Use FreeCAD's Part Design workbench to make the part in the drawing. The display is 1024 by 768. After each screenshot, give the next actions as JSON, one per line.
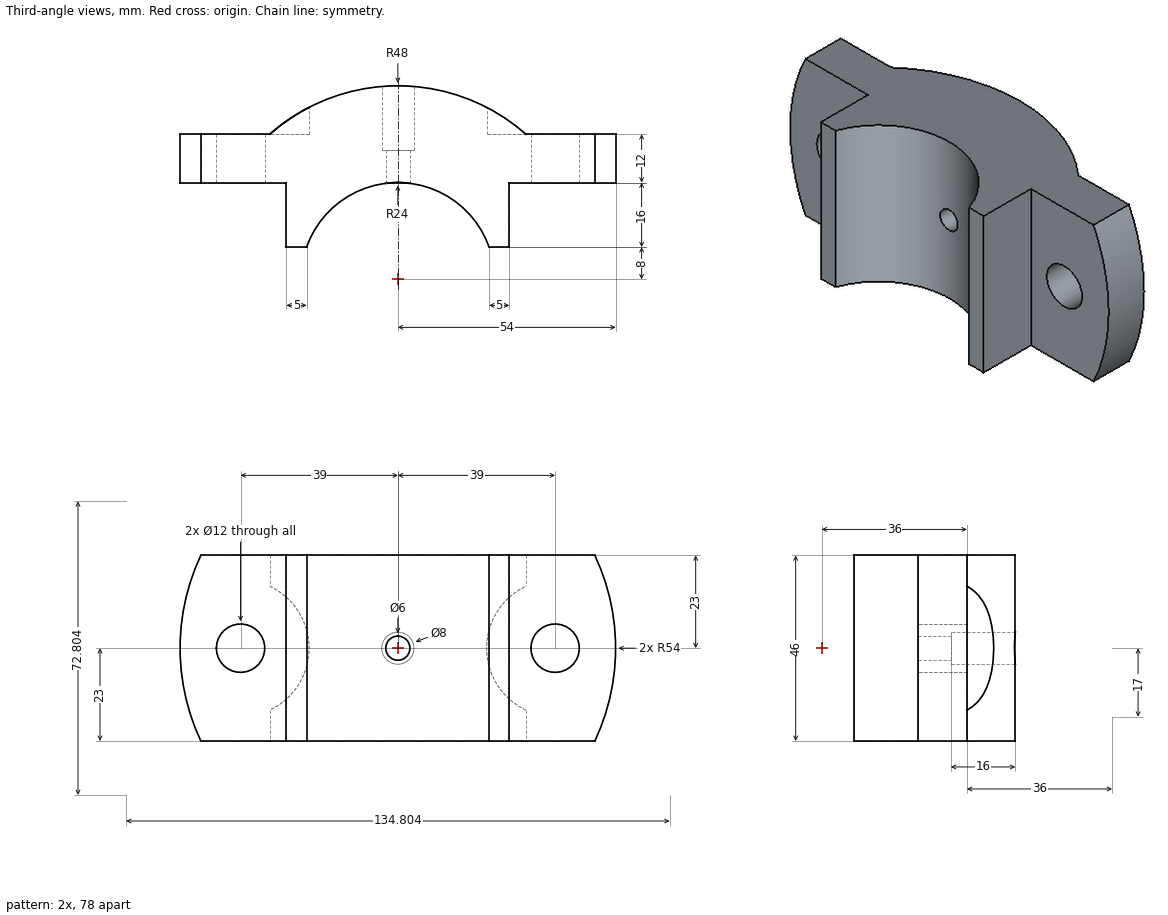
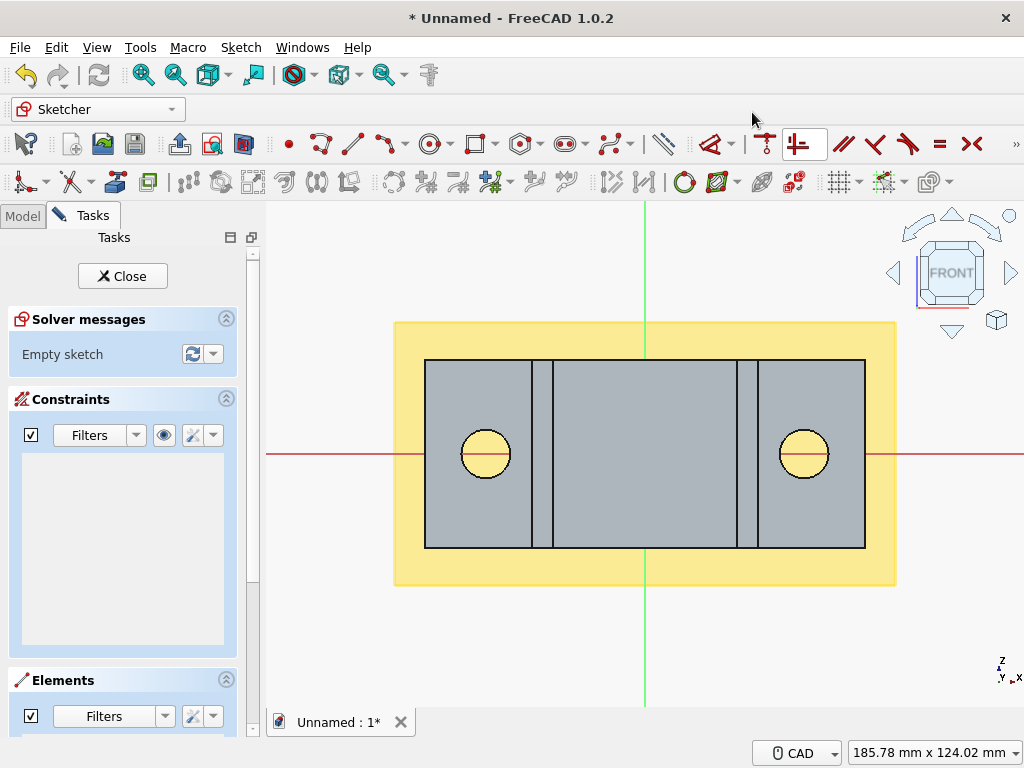
{"action": "left_click", "coordinate": [244, 144]}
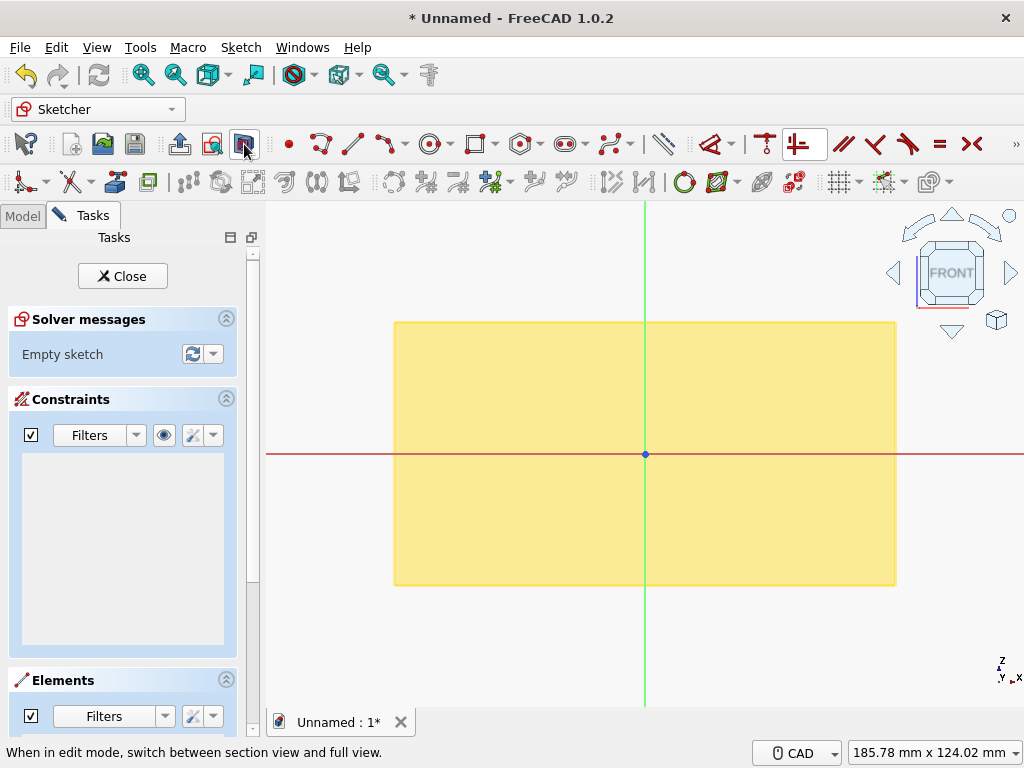
{"action": "scroll", "coordinate": [650, 454], "scroll_direction": "up", "scroll_amount": 13}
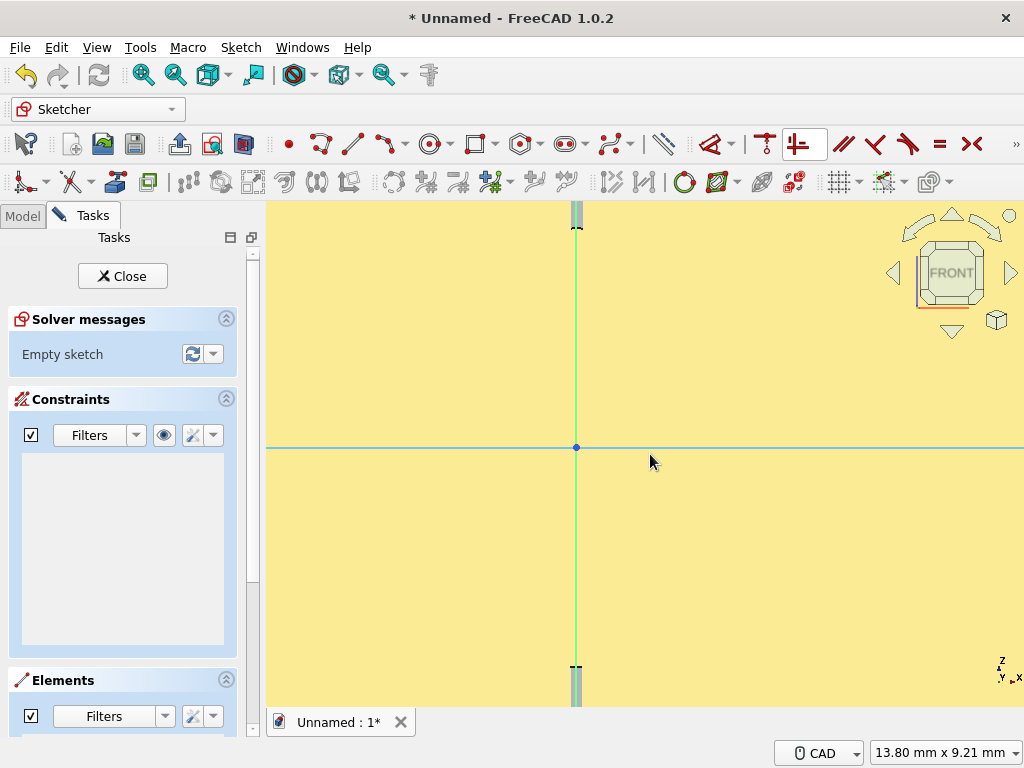
{"action": "left_click", "coordinate": [430, 144]}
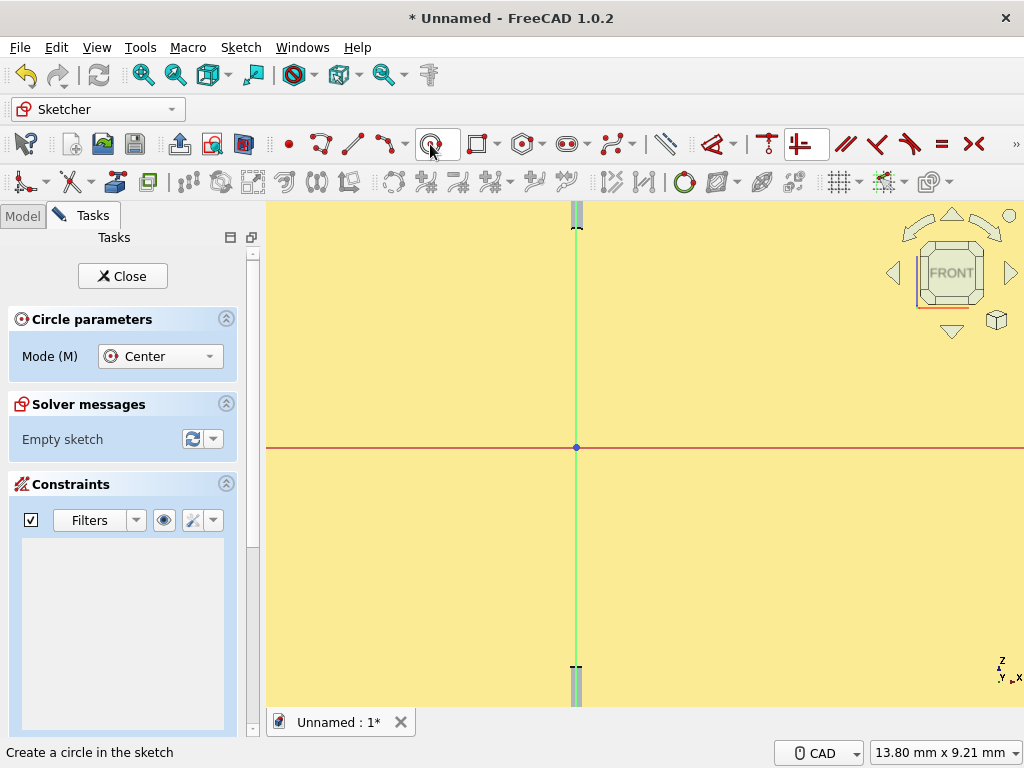
{"action": "left_click", "coordinate": [576, 448]}
{"action": "mouse_move", "coordinate": [693, 331]}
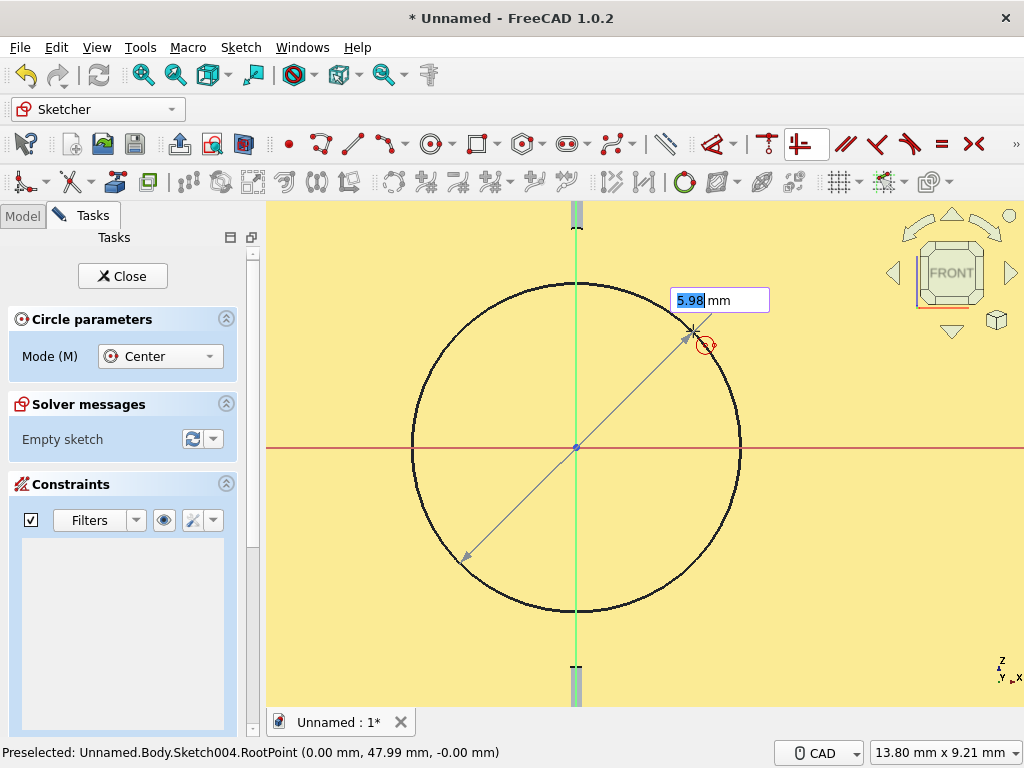
{"action": "type", "text": "6"}
{"action": "key", "text": "Return"}
{"action": "key", "text": "Escape"}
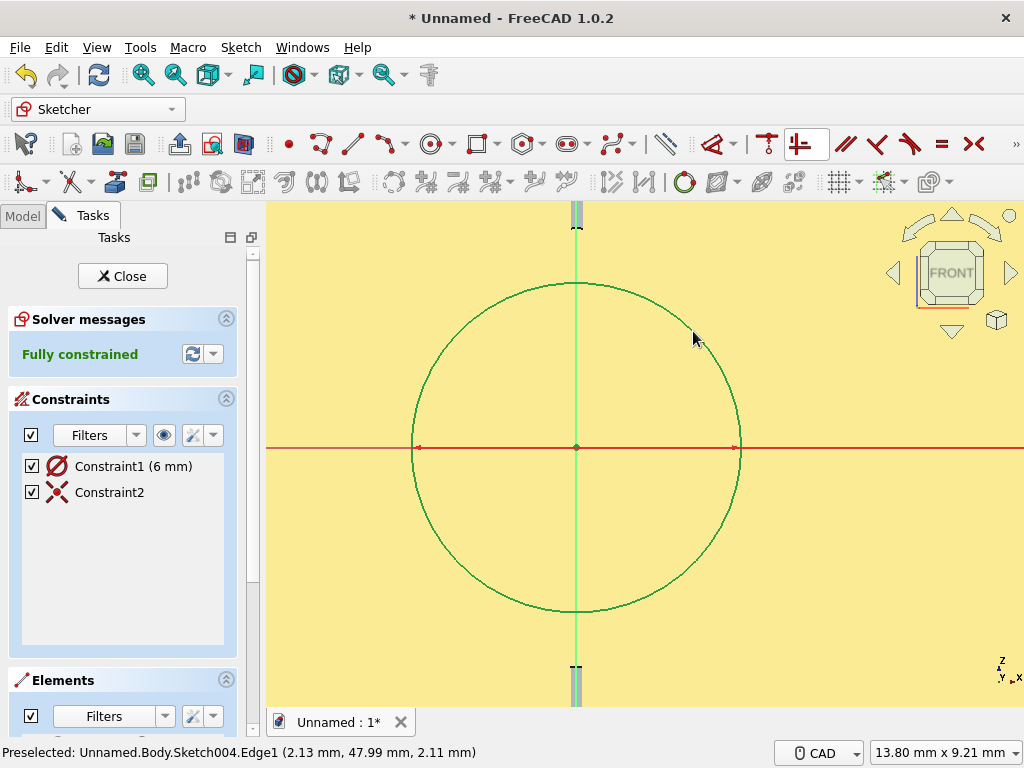
{"action": "left_click", "coordinate": [123, 276]}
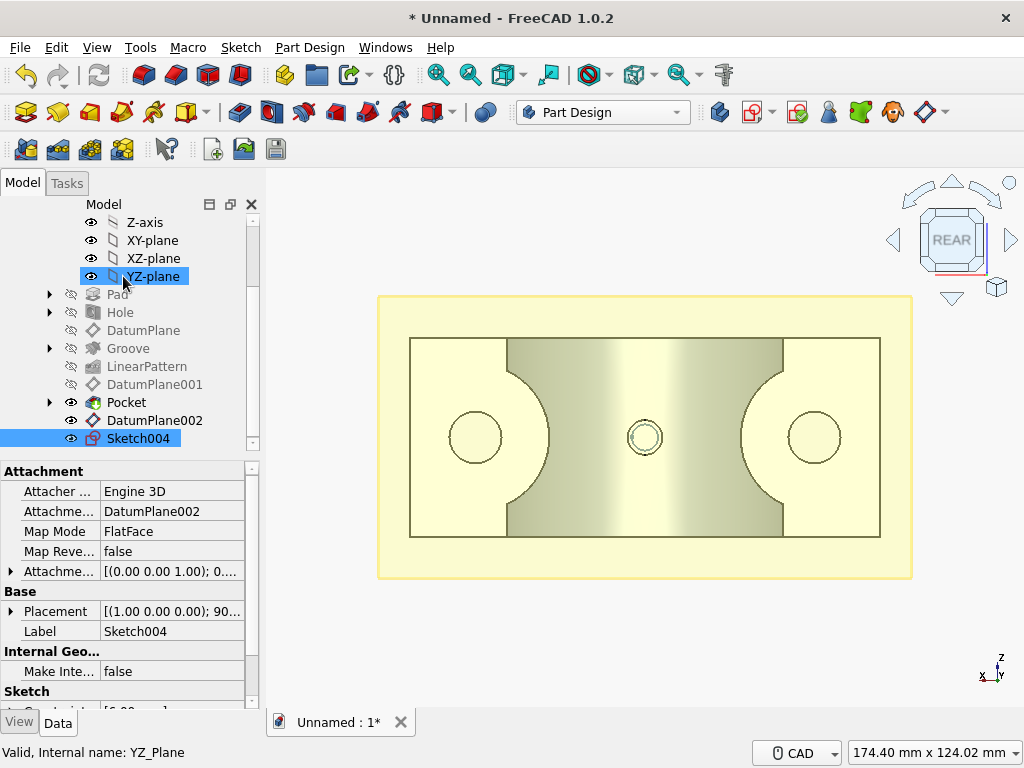
{"action": "left_click", "coordinate": [240, 112]}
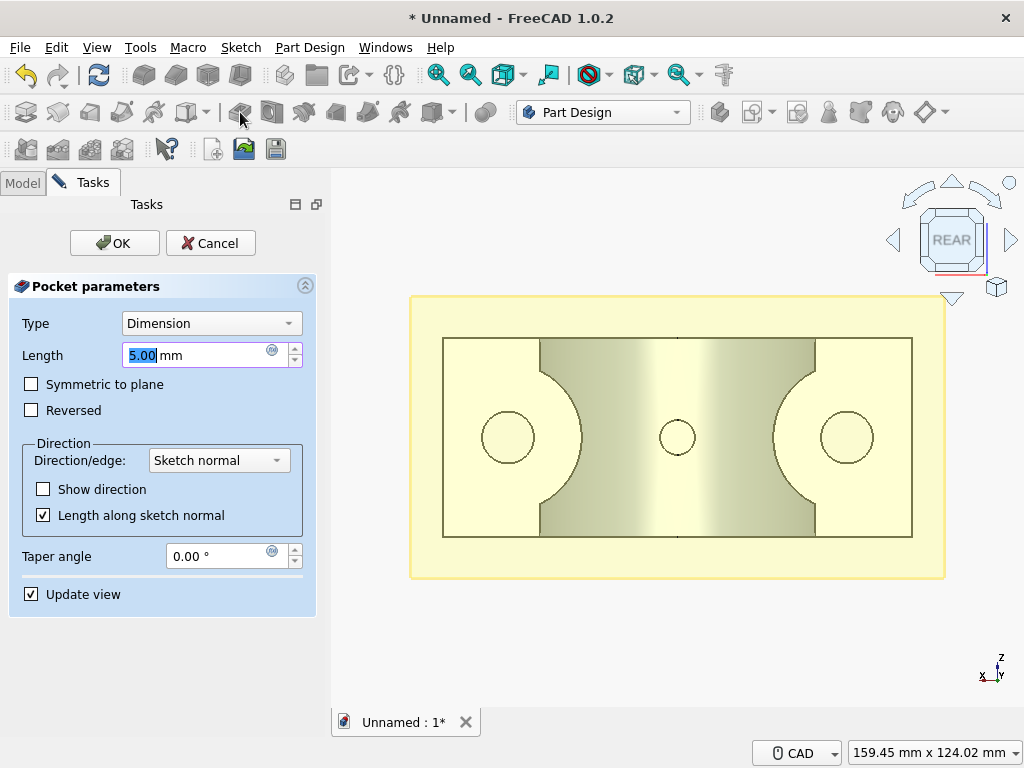
{"action": "left_click", "coordinate": [212, 324]}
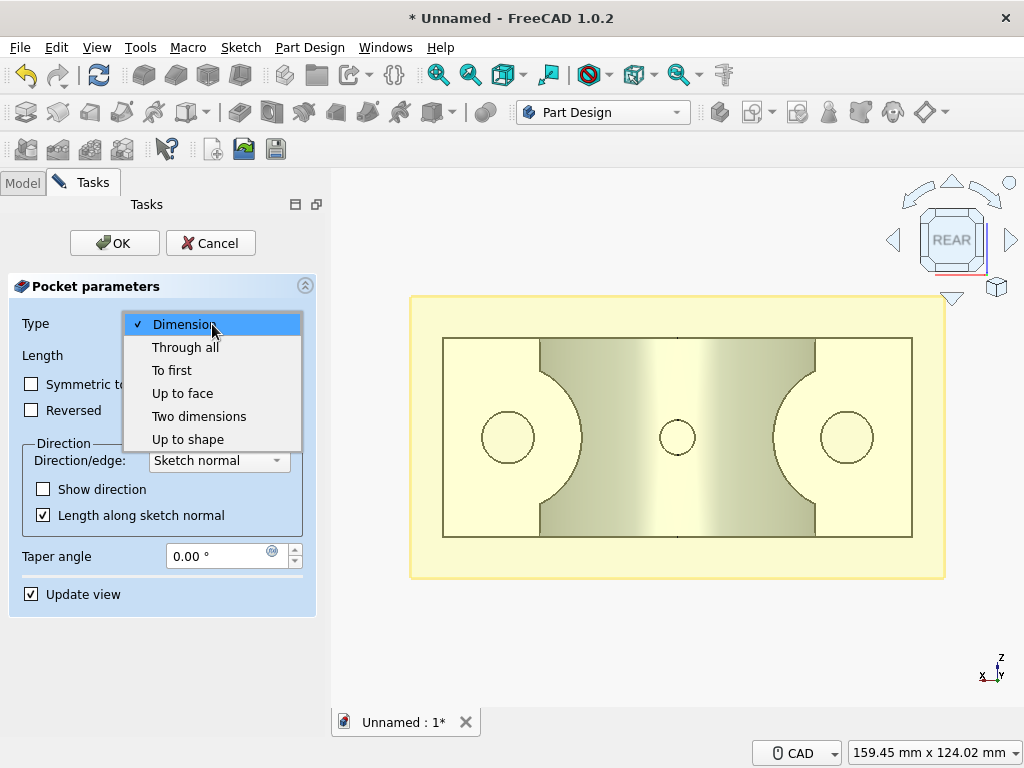
{"action": "left_click", "coordinate": [212, 348]}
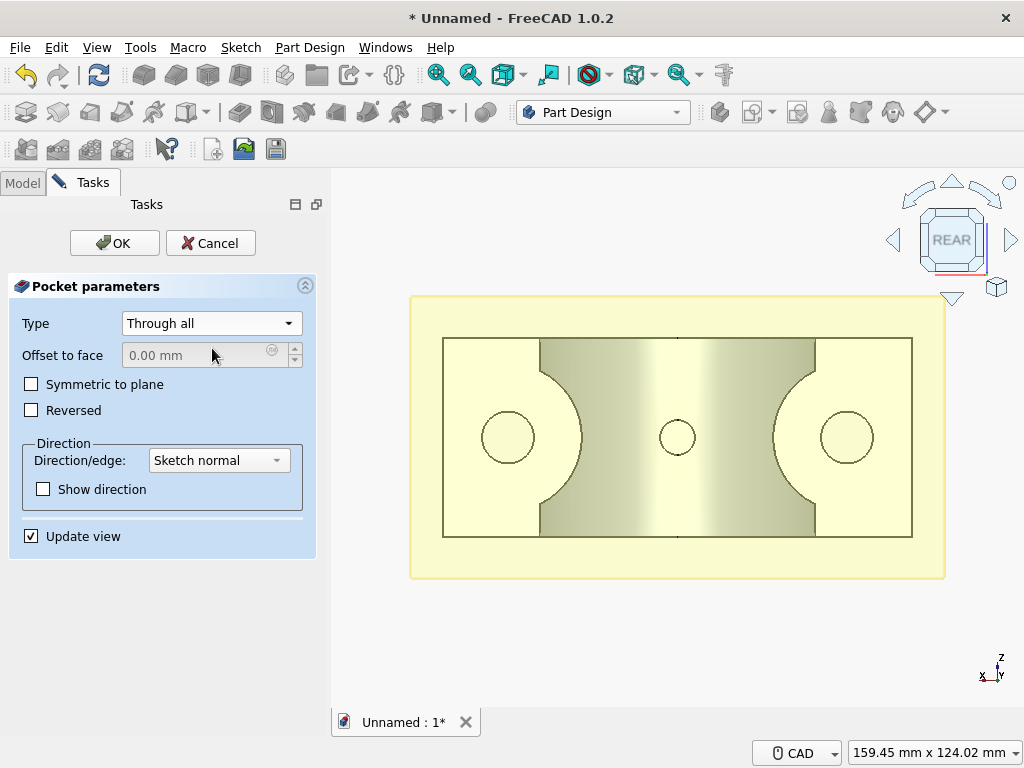
{"action": "left_click", "coordinate": [30, 410]}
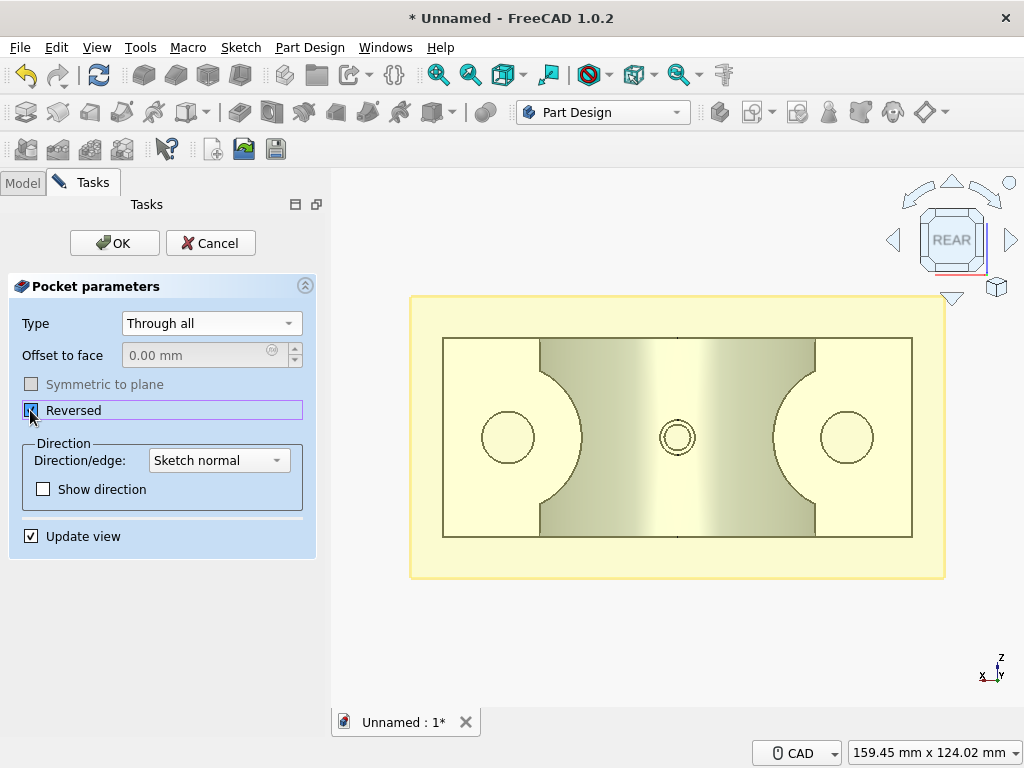
{"action": "left_click", "coordinate": [115, 243]}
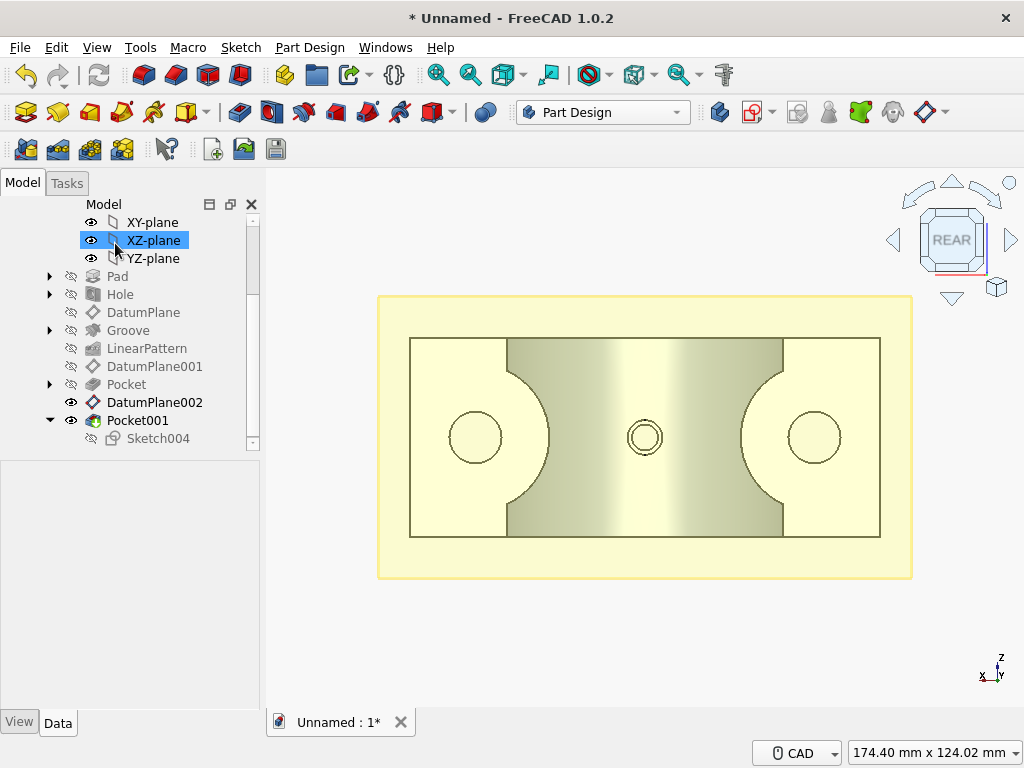
{"action": "left_click", "coordinate": [116, 402]}
{"action": "key", "text": "space"}